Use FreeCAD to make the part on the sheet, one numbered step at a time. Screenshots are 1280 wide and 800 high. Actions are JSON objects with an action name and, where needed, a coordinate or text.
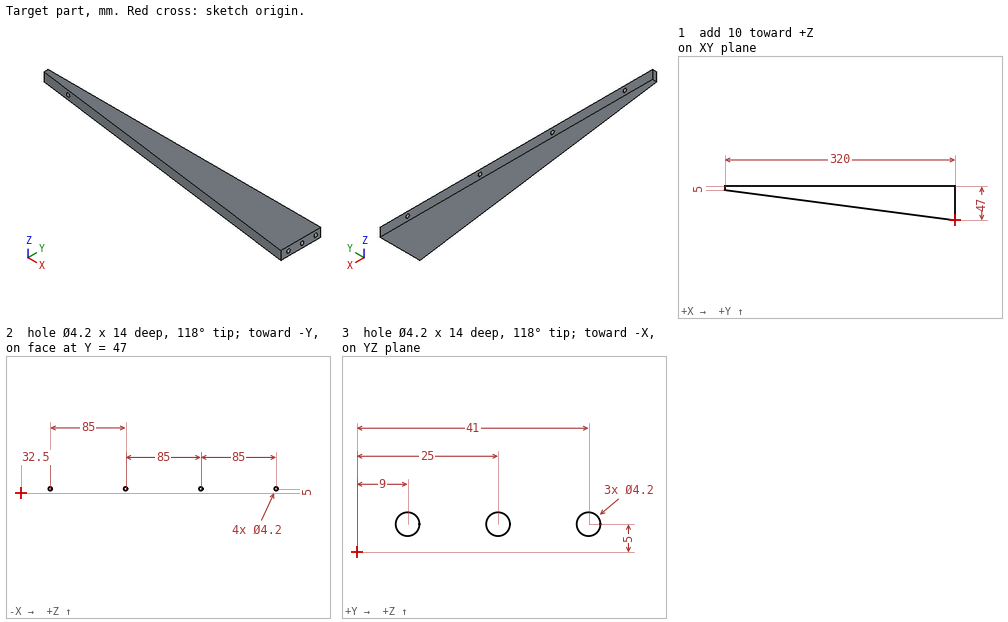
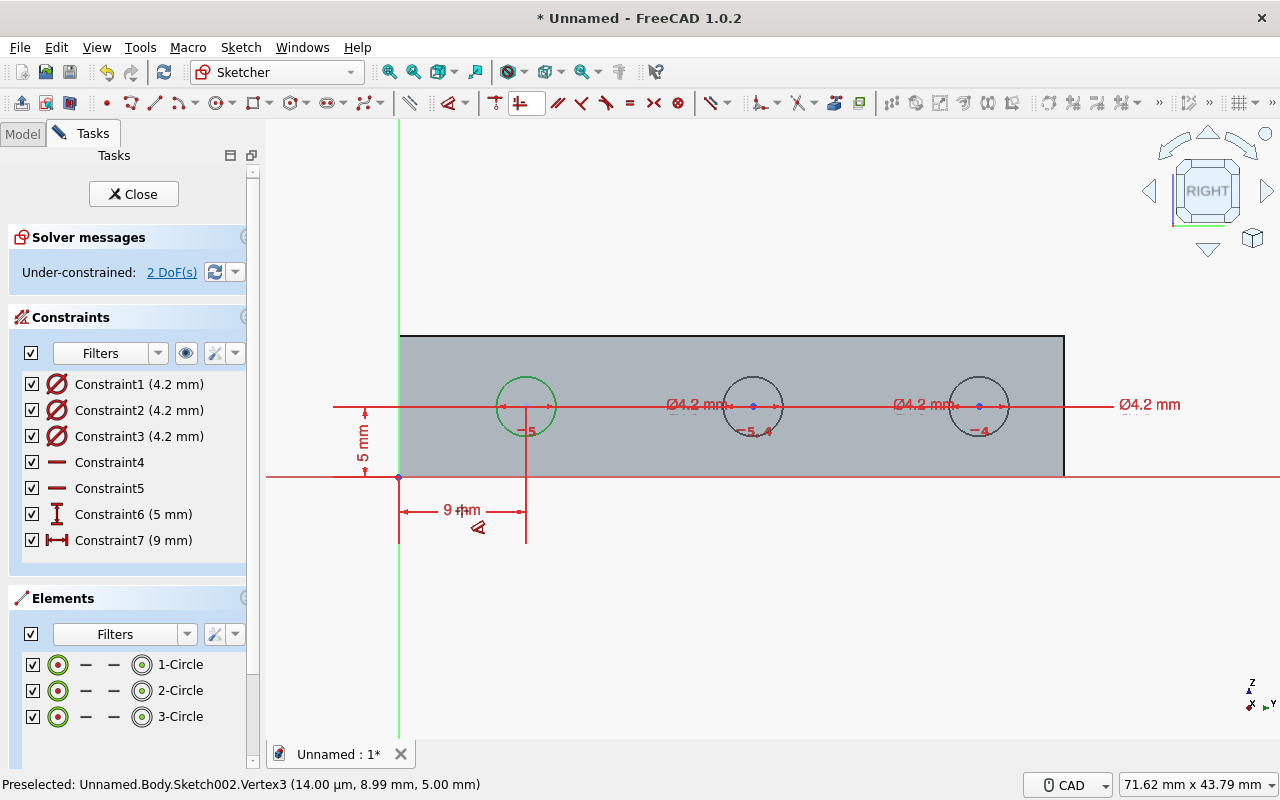
{"action": "left_click", "coordinate": [979, 407]}
{"action": "left_click", "coordinate": [689, 511]}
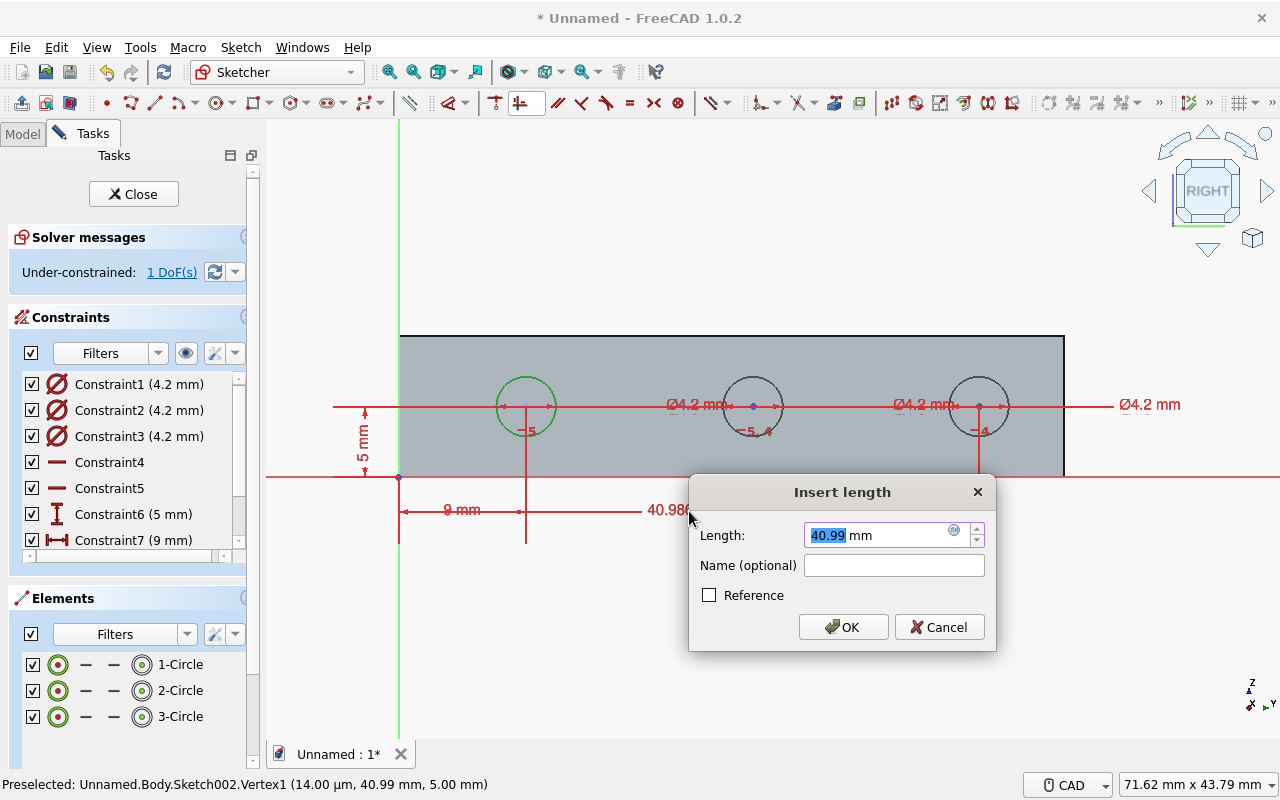
{"action": "type", "text": "41"}
{"action": "key", "text": "Return"}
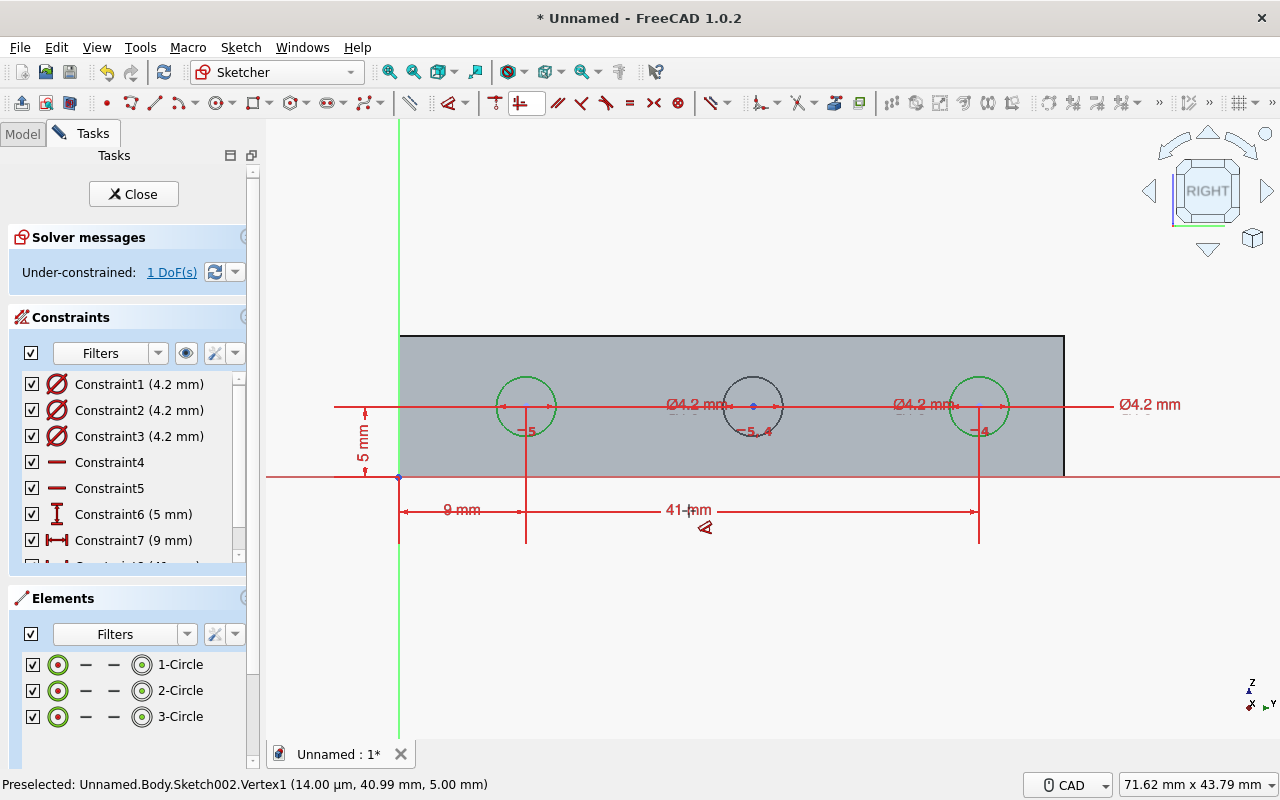
{"action": "left_click", "coordinate": [753, 407]}
{"action": "left_click", "coordinate": [576, 511]}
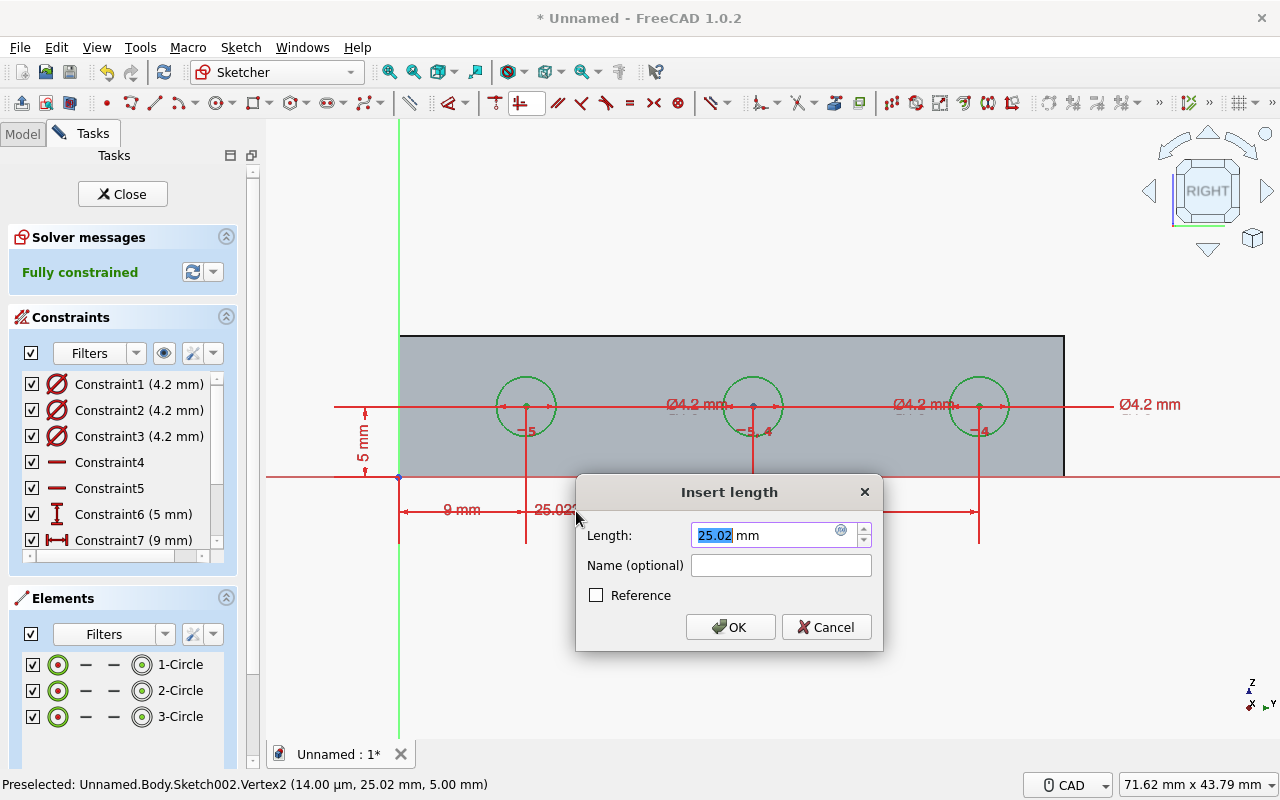
{"action": "type", "text": "25"}
{"action": "key", "text": "Return"}
{"action": "key", "text": "Escape"}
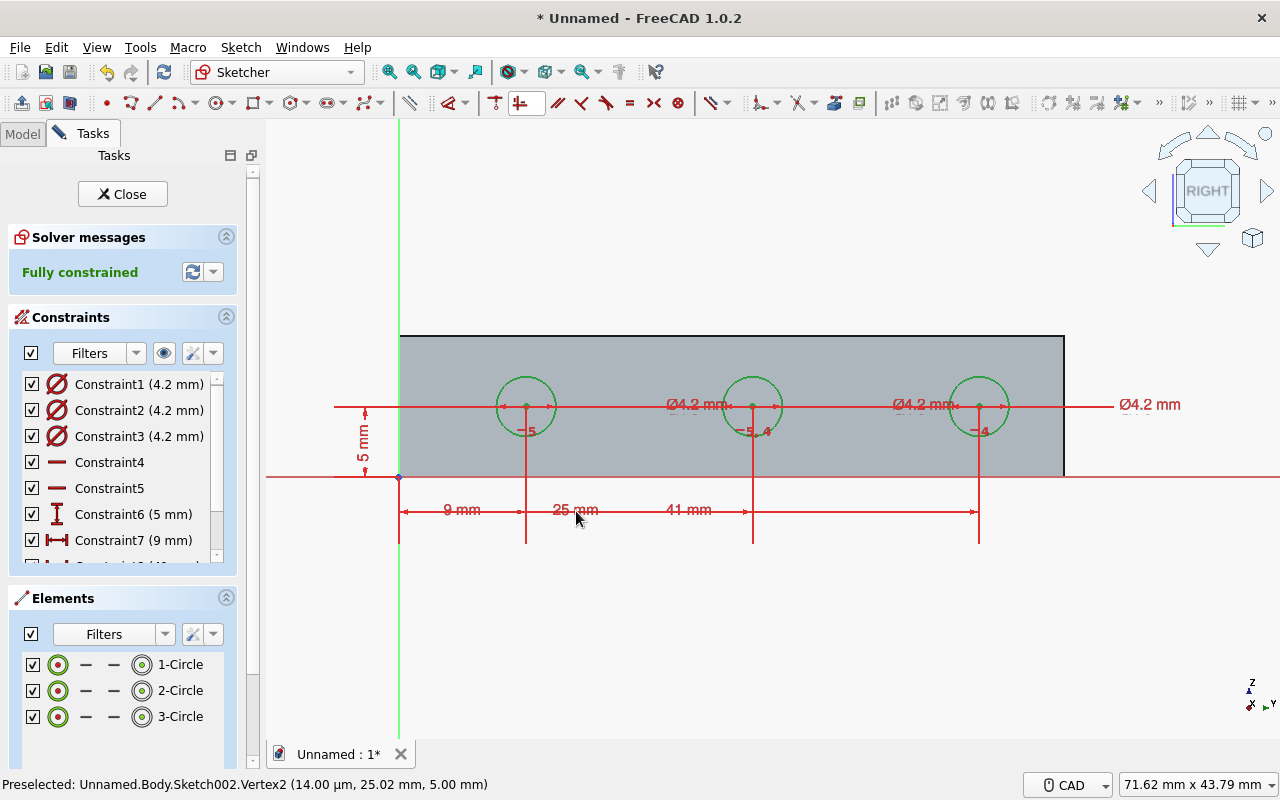
{"action": "left_click", "coordinate": [123, 194]}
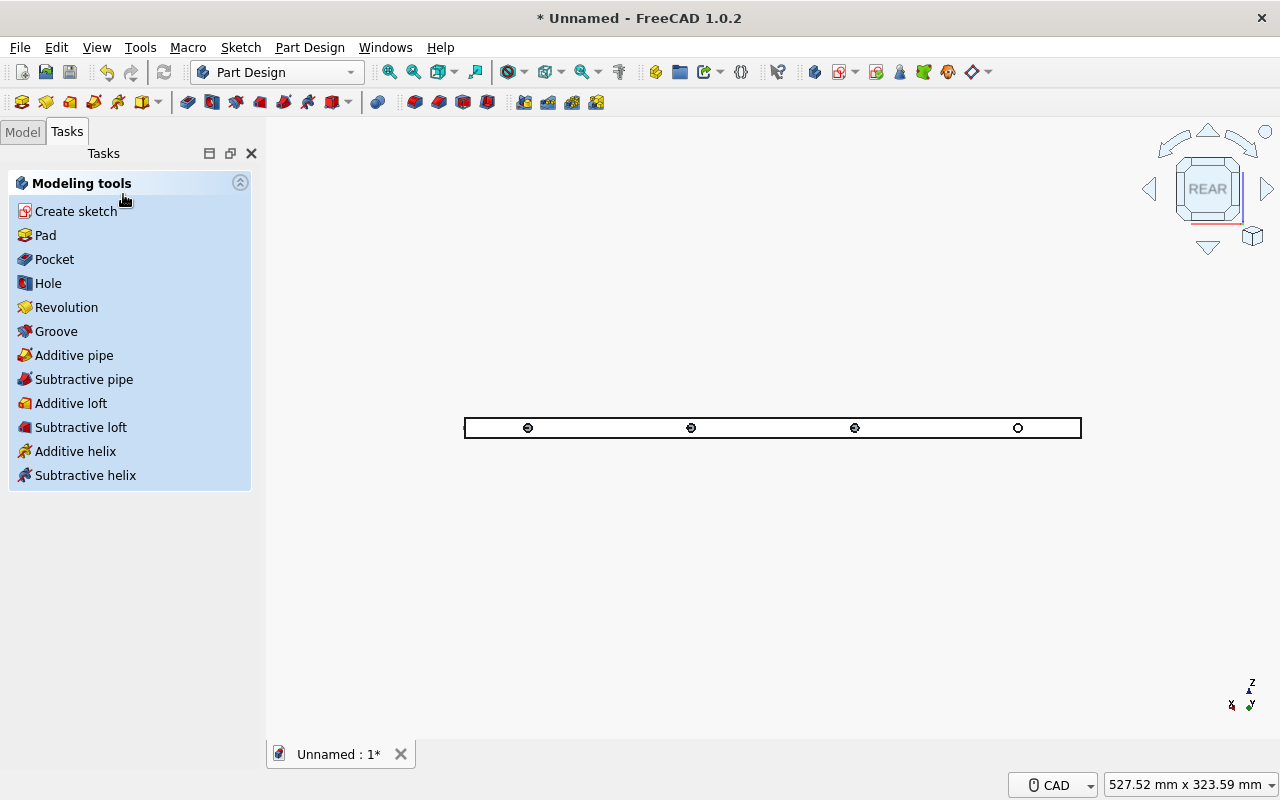
{"action": "left_click", "coordinate": [212, 102]}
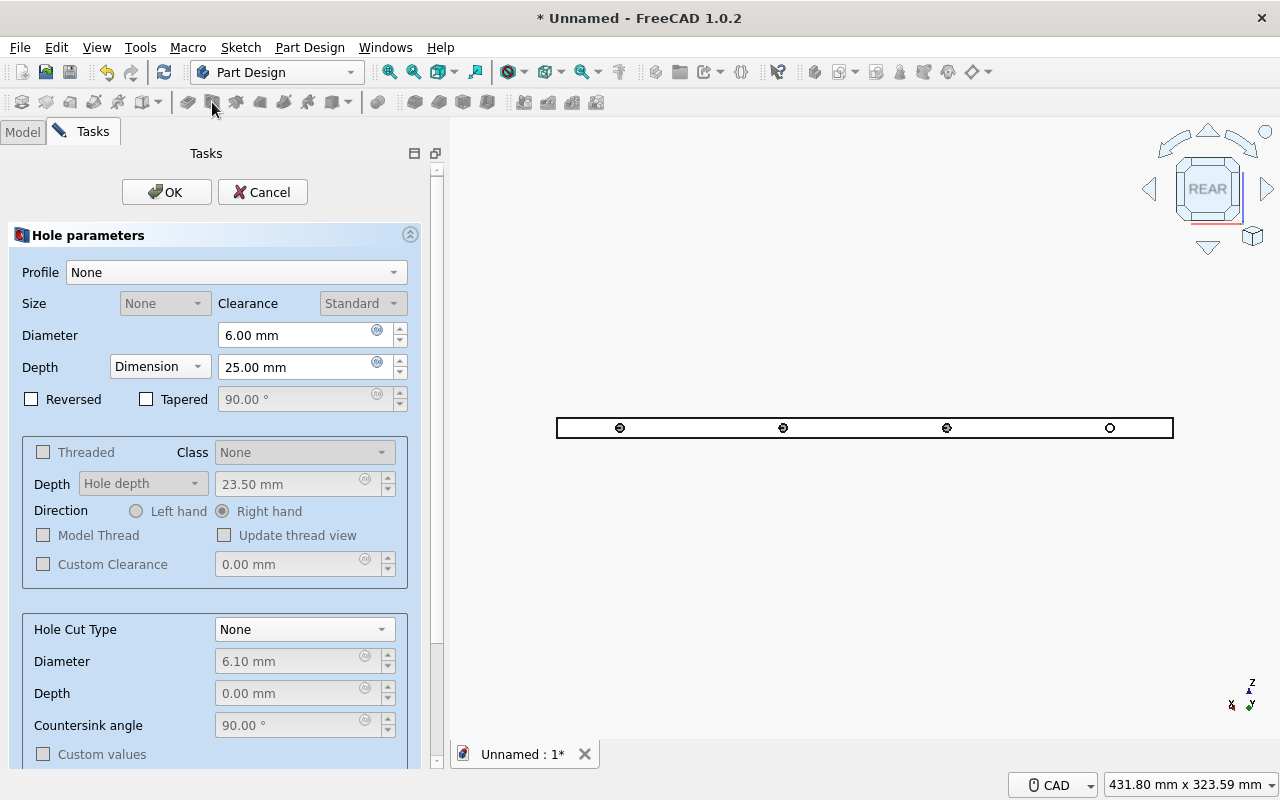
{"action": "triple_click", "coordinate": [305, 335]}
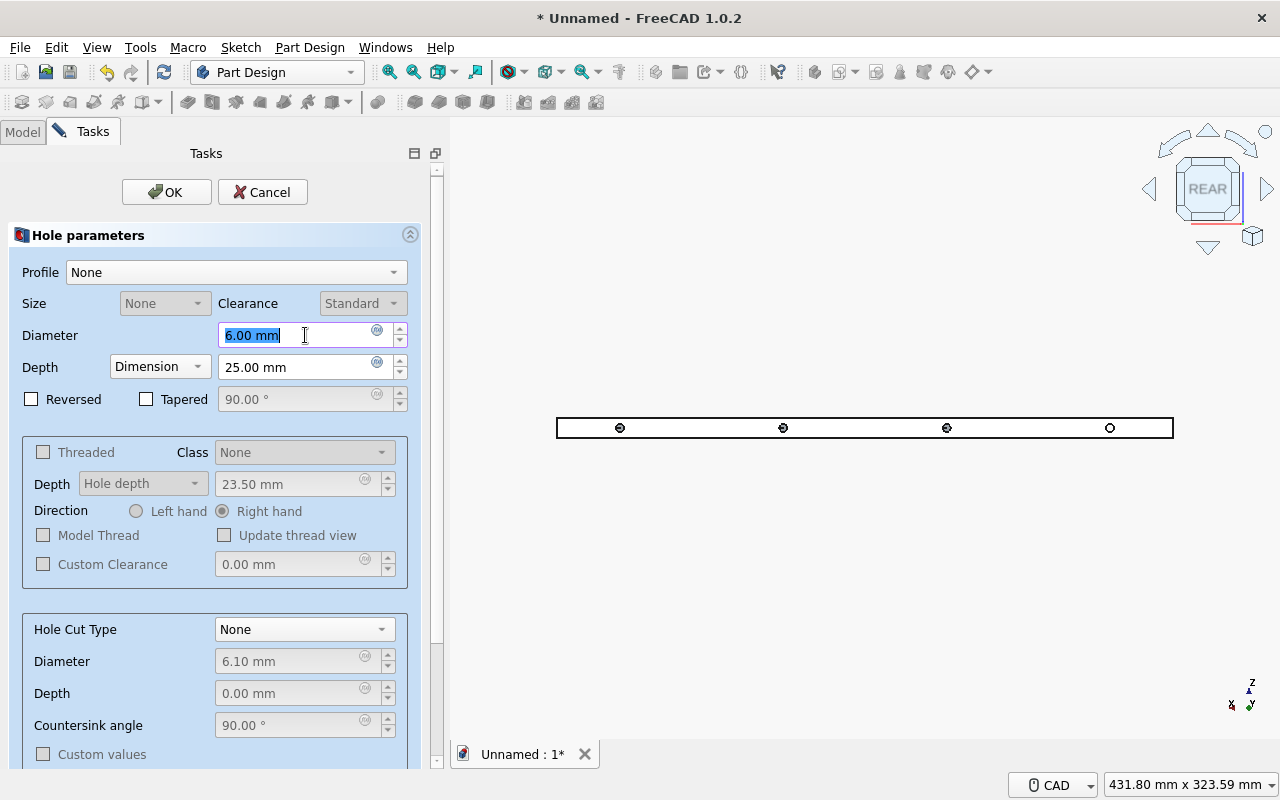
{"action": "type", "text": "4.2"}
{"action": "key", "text": "Tab"}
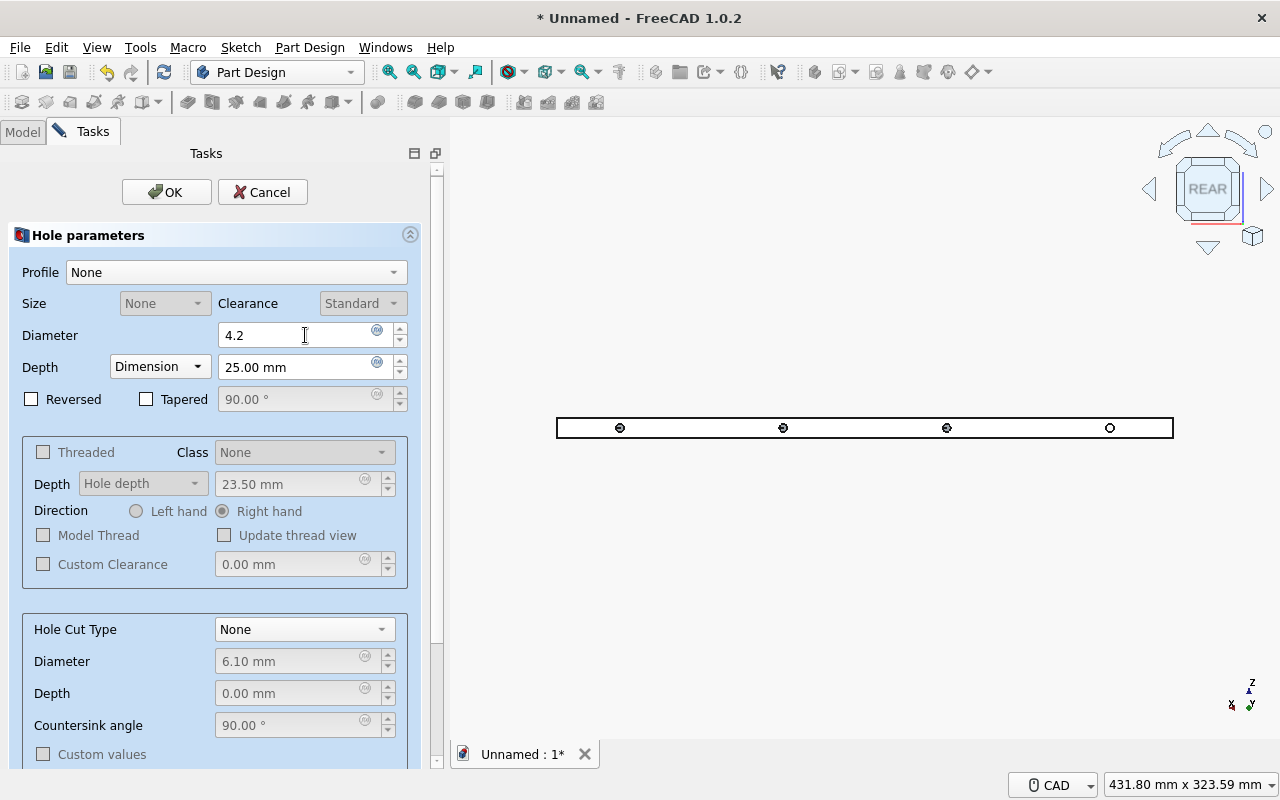
{"action": "triple_click", "coordinate": [305, 367]}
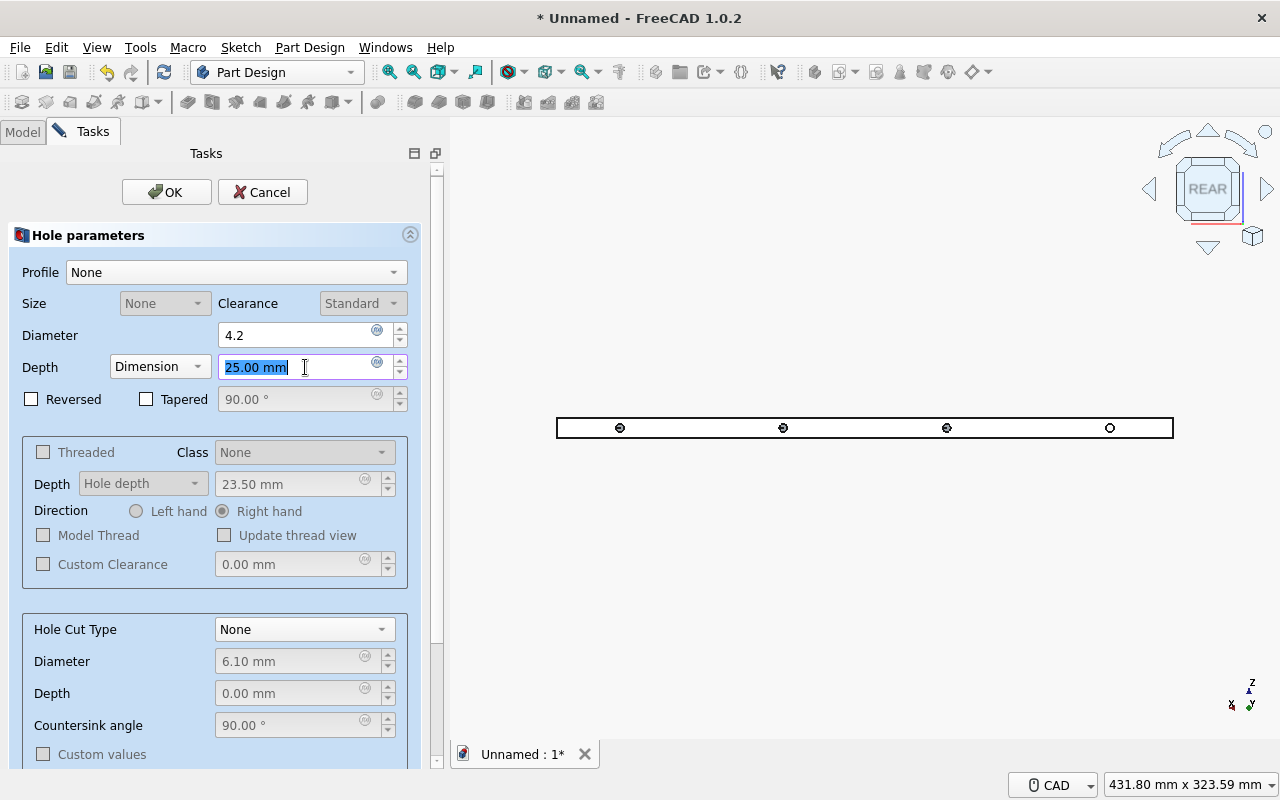
{"action": "type", "text": "14"}
{"action": "key", "text": "Tab"}